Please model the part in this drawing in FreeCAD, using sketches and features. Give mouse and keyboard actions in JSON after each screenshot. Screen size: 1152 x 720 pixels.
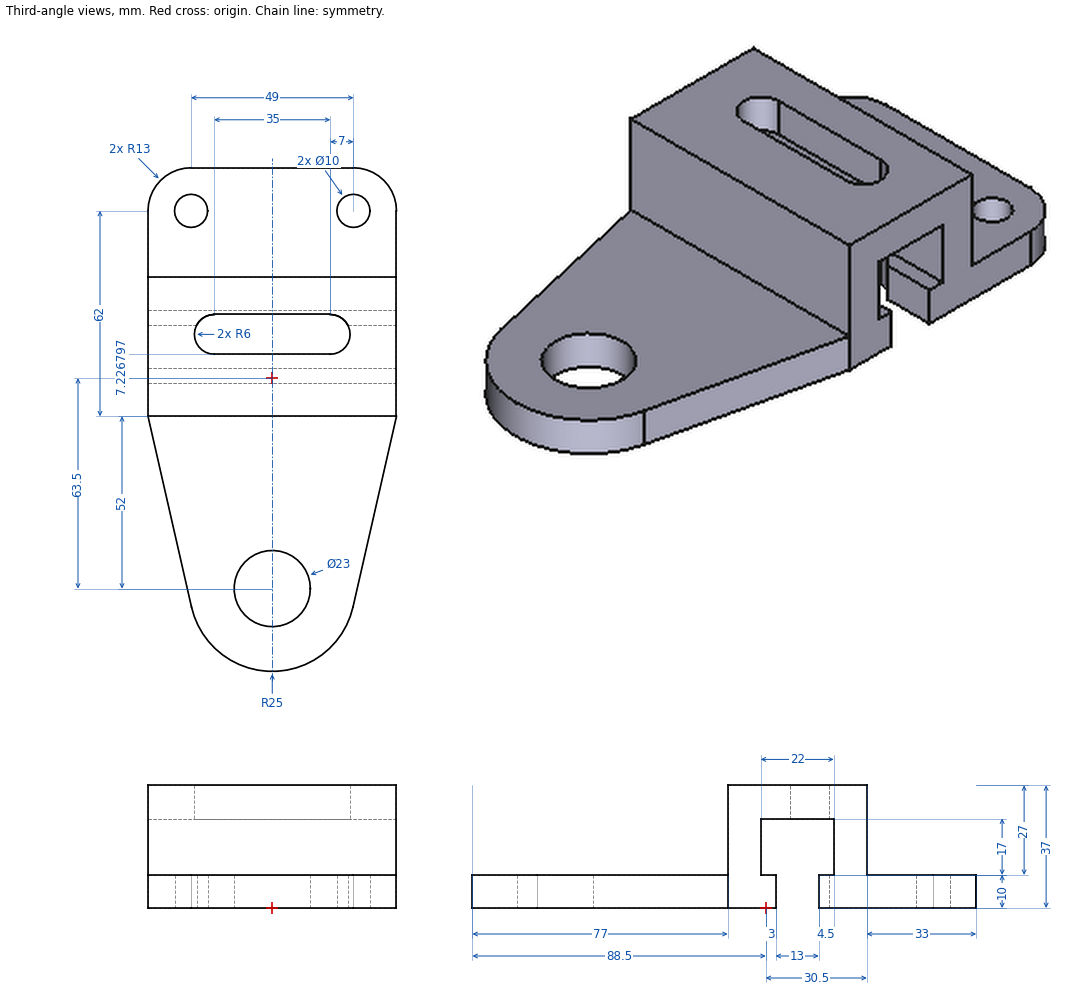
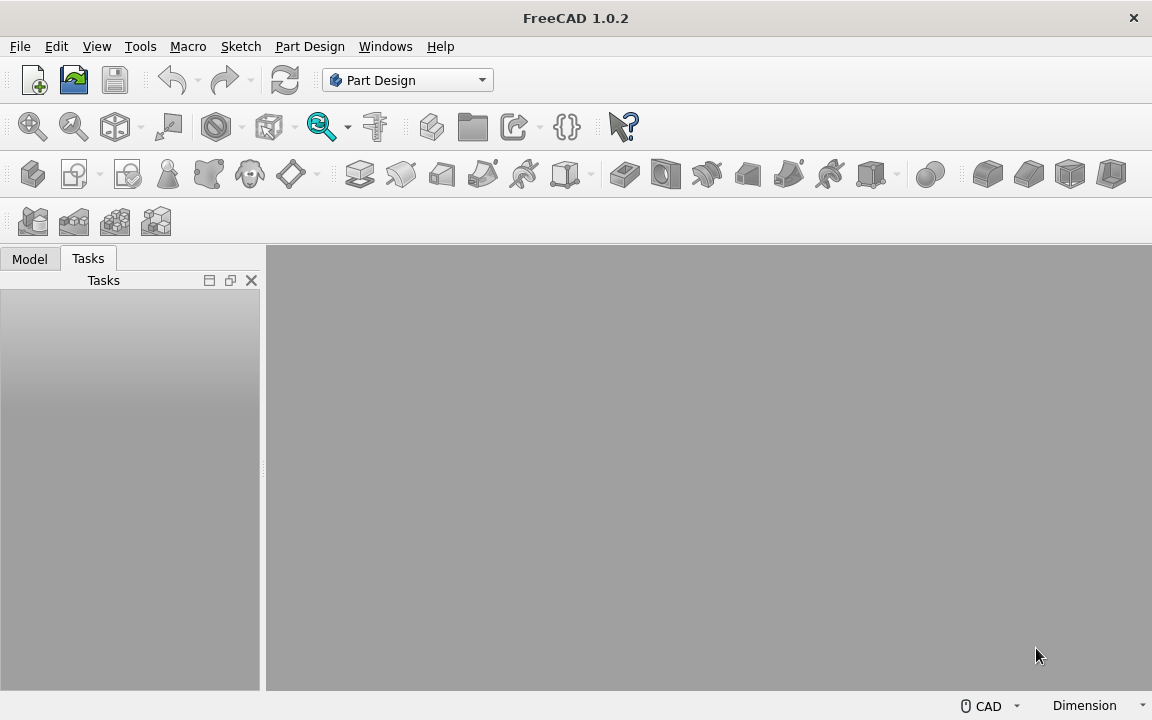
{"action": "left_click", "coordinate": [33, 80]}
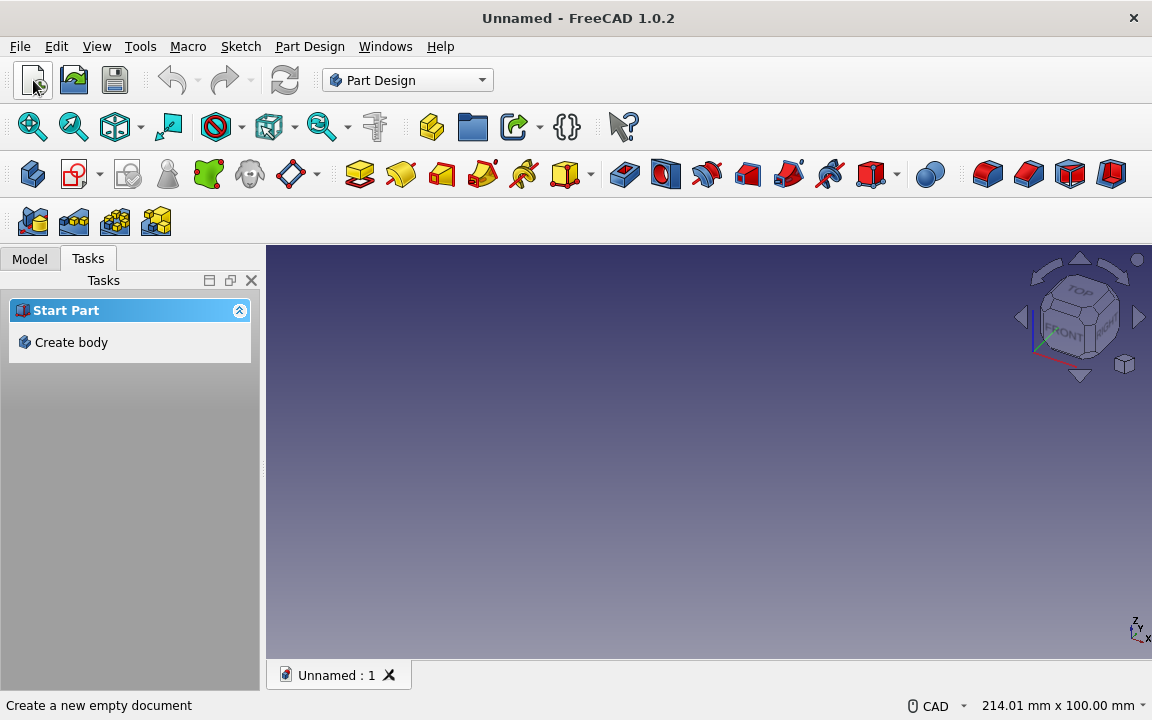
{"action": "left_click", "coordinate": [74, 174]}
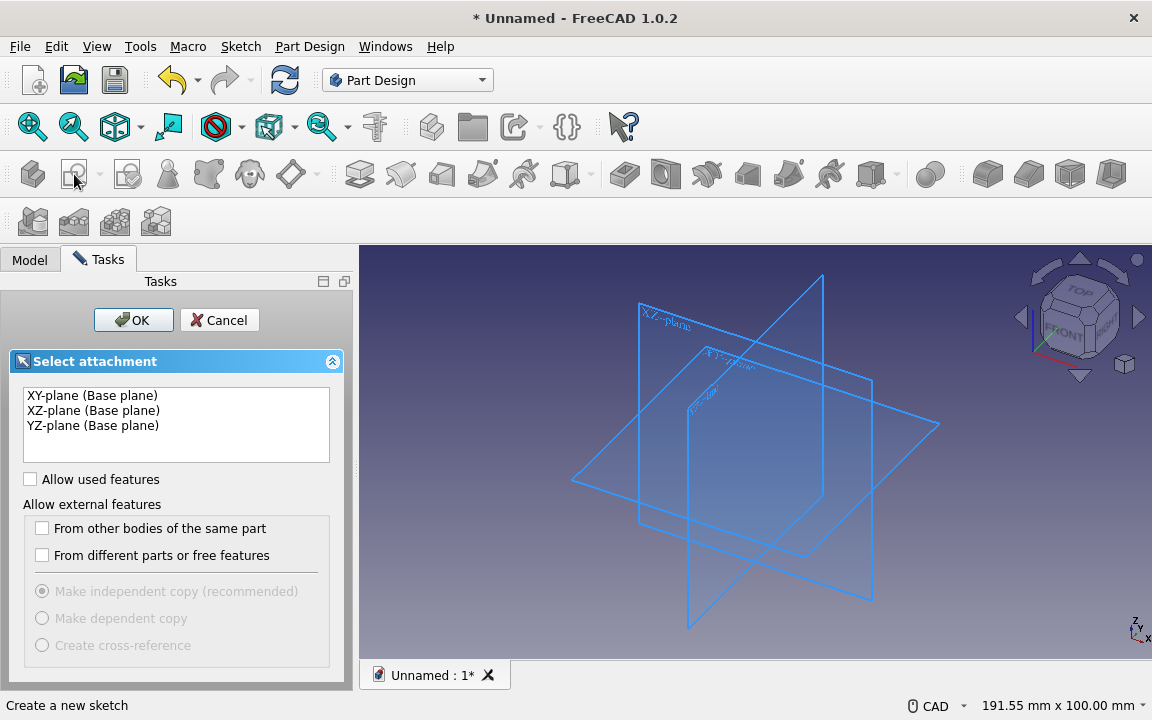
{"action": "left_click", "coordinate": [84, 396]}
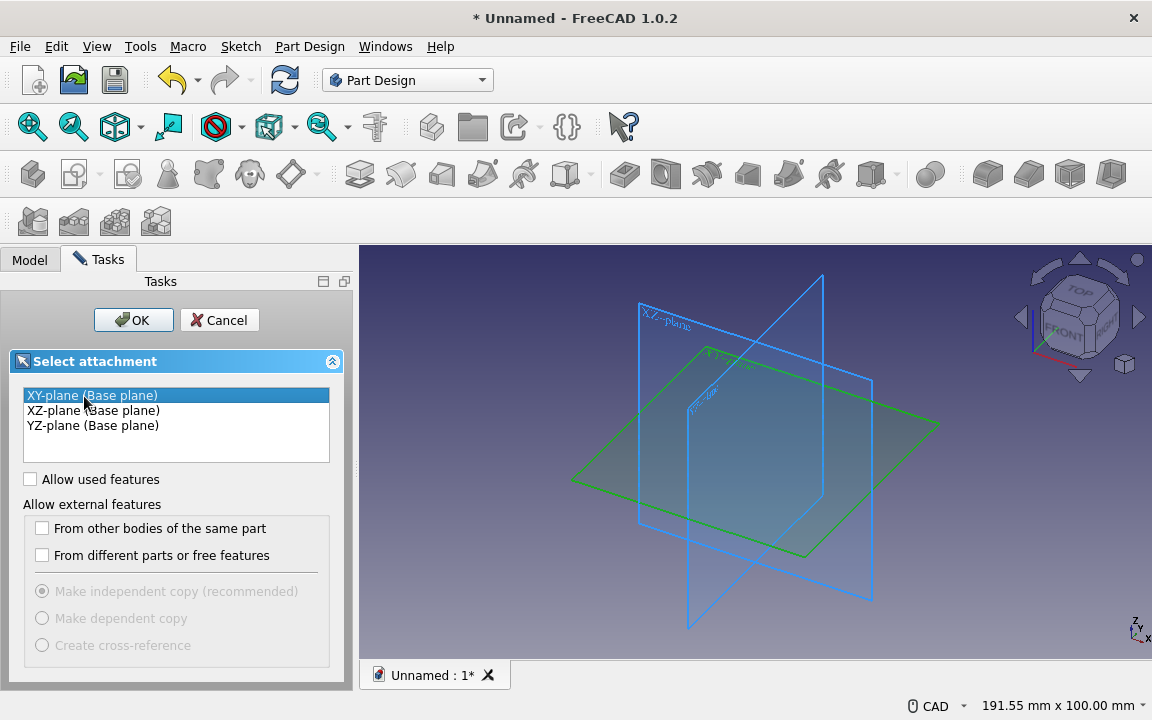
{"action": "left_click", "coordinate": [134, 320]}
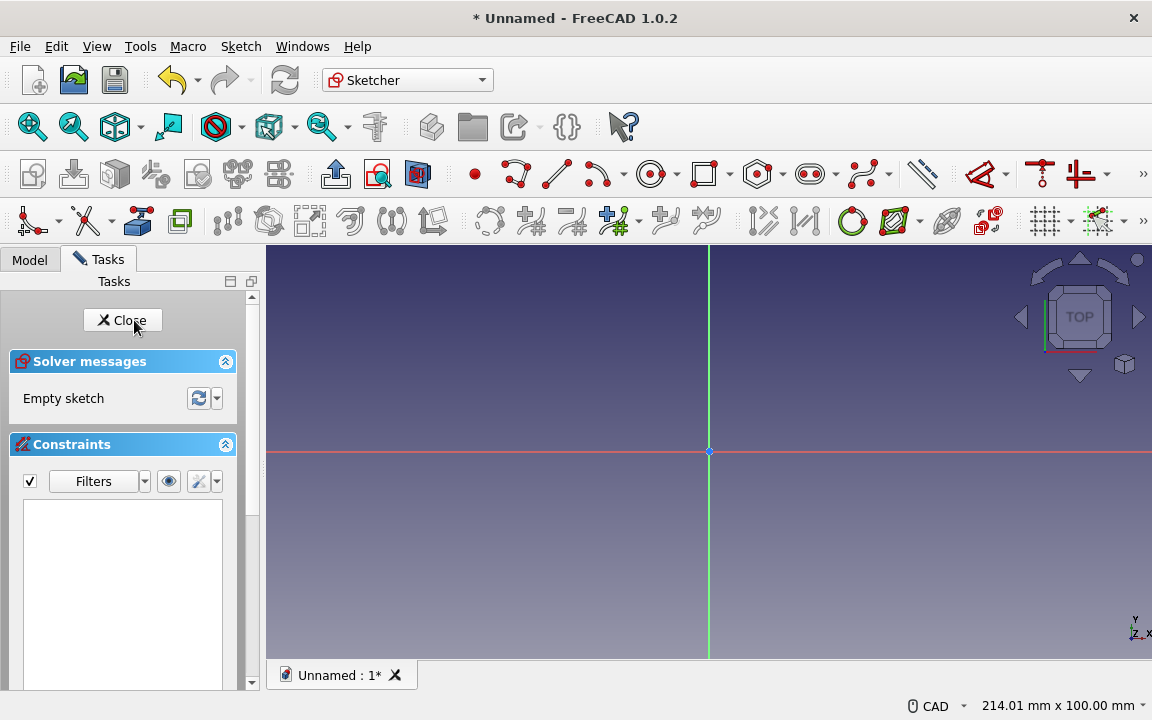
{"action": "scroll", "coordinate": [601, 422], "scroll_direction": "down", "scroll_amount": 5}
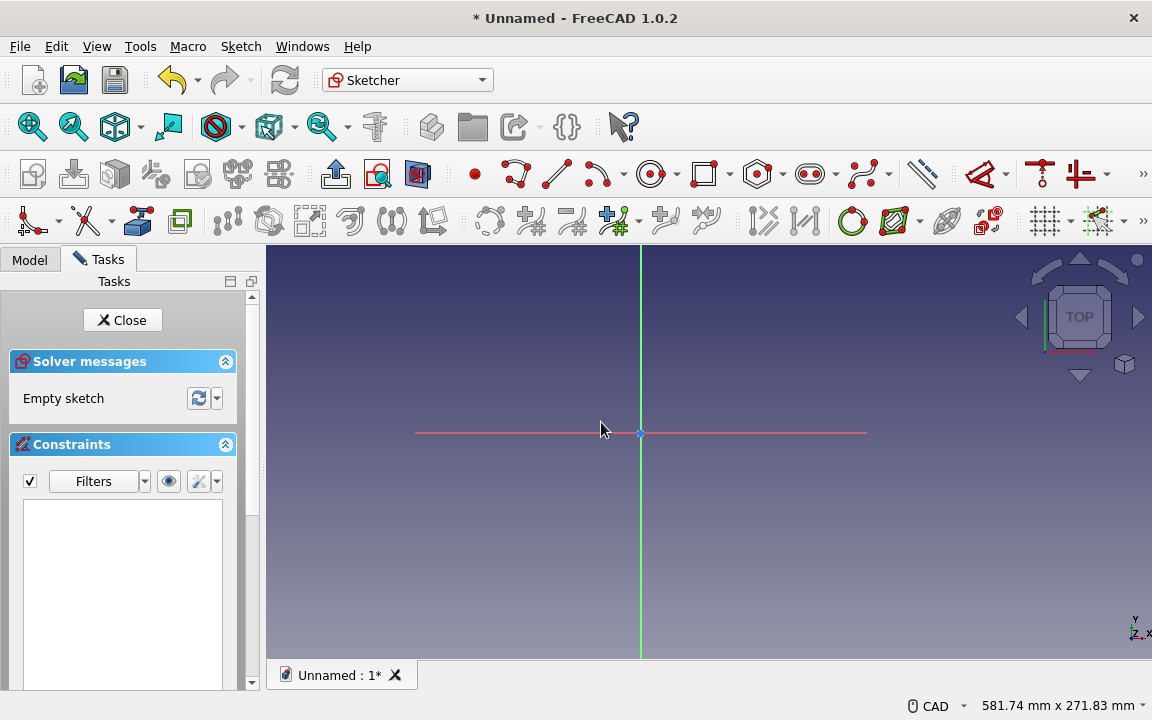
{"action": "left_click", "coordinate": [557, 174]}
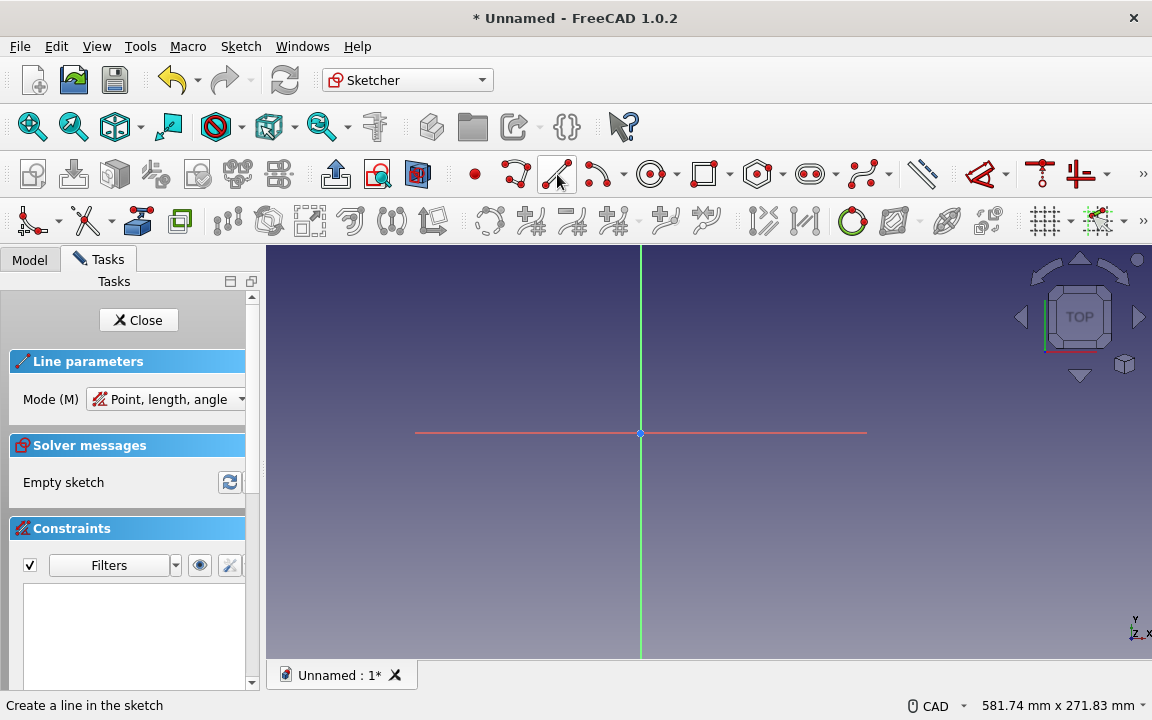
{"action": "left_click", "coordinate": [678, 337]}
{"action": "left_click", "coordinate": [604, 337]}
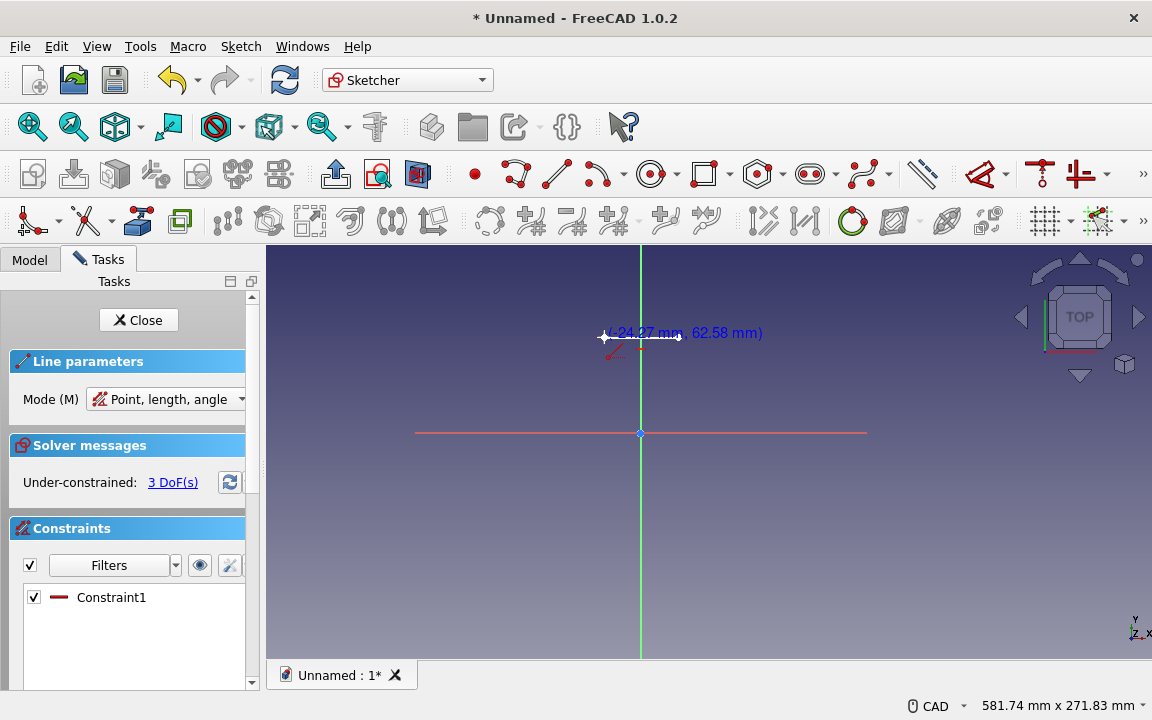
{"action": "left_click", "coordinate": [516, 174]}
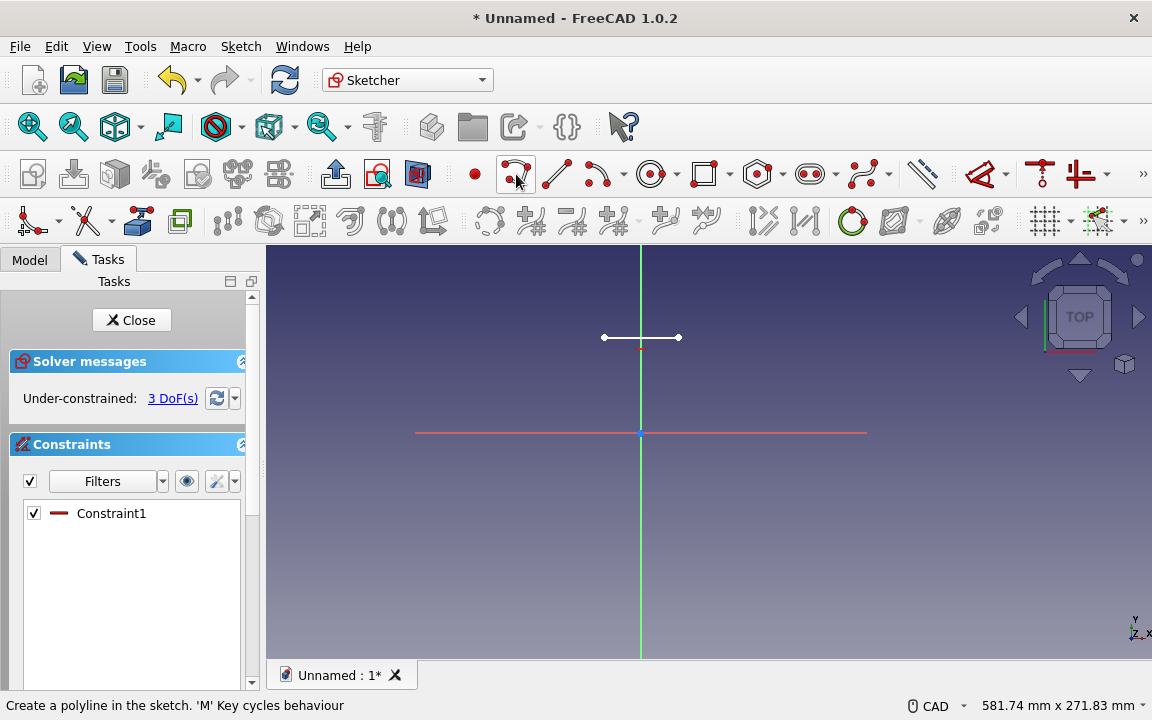
{"action": "left_click", "coordinate": [584, 356]}
{"action": "left_click", "coordinate": [584, 451]}
{"action": "left_click", "coordinate": [604, 538]}
{"action": "right_click", "coordinate": [604, 538]}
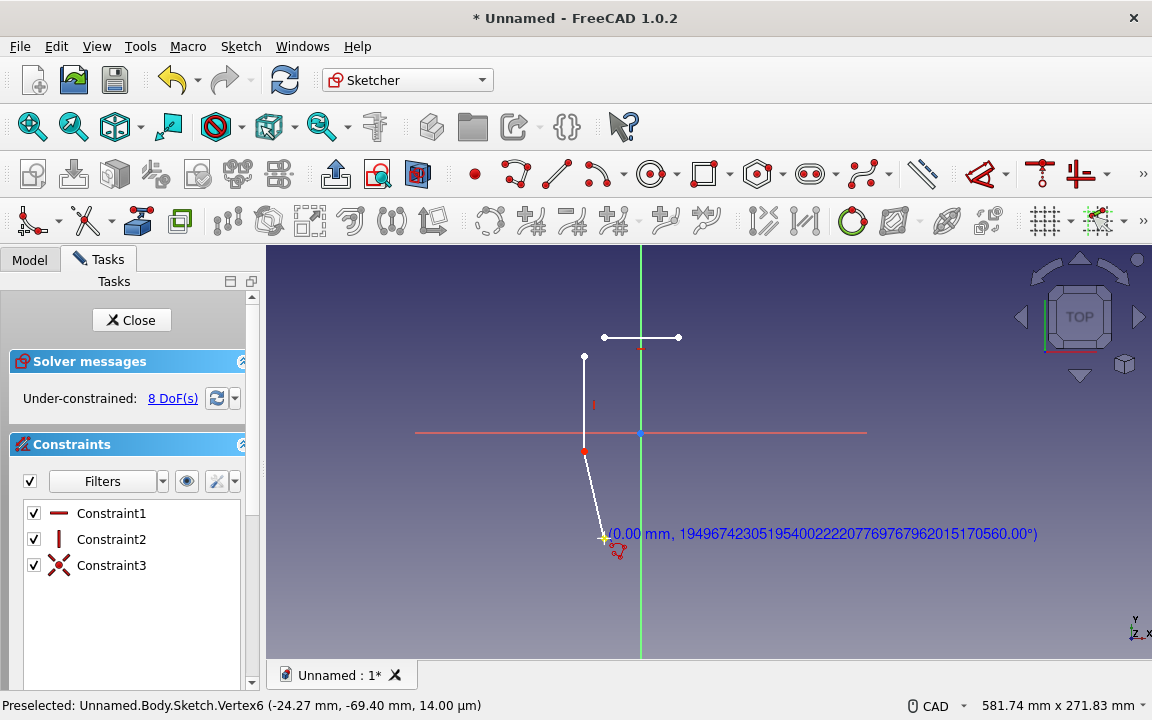
{"action": "left_click", "coordinate": [678, 538]}
{"action": "left_click", "coordinate": [698, 451]}
{"action": "left_click", "coordinate": [698, 356]}
{"action": "right_click", "coordinate": [698, 356]}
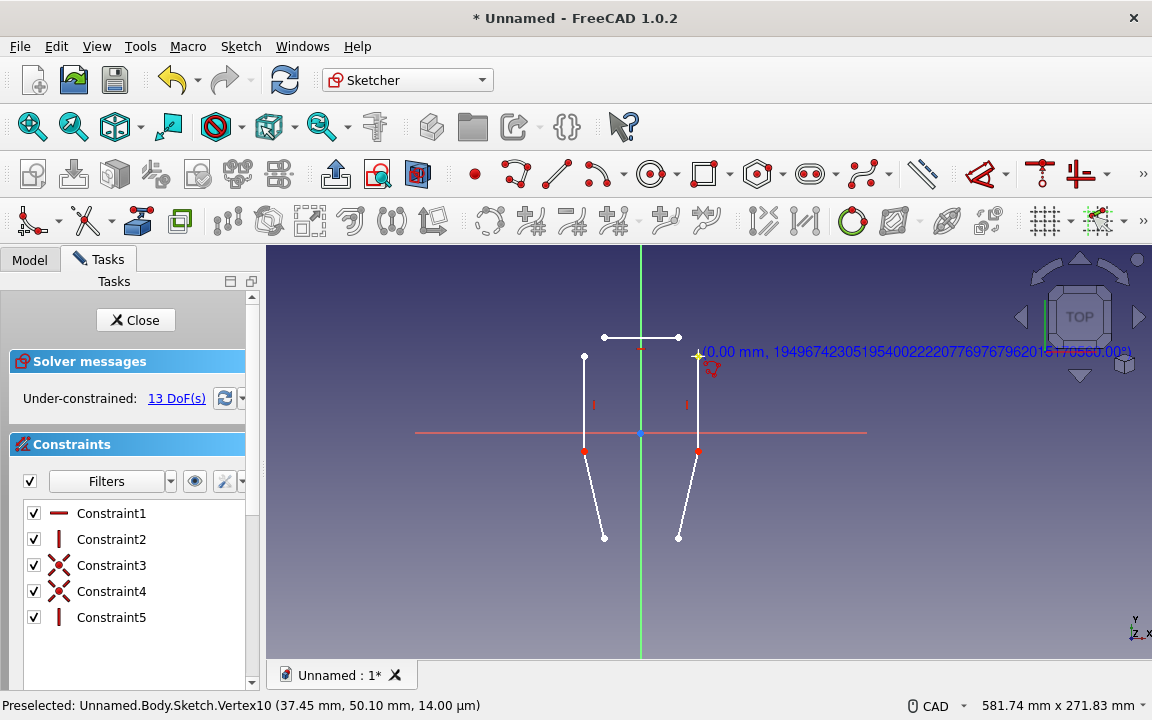
{"action": "left_click", "coordinate": [624, 174]}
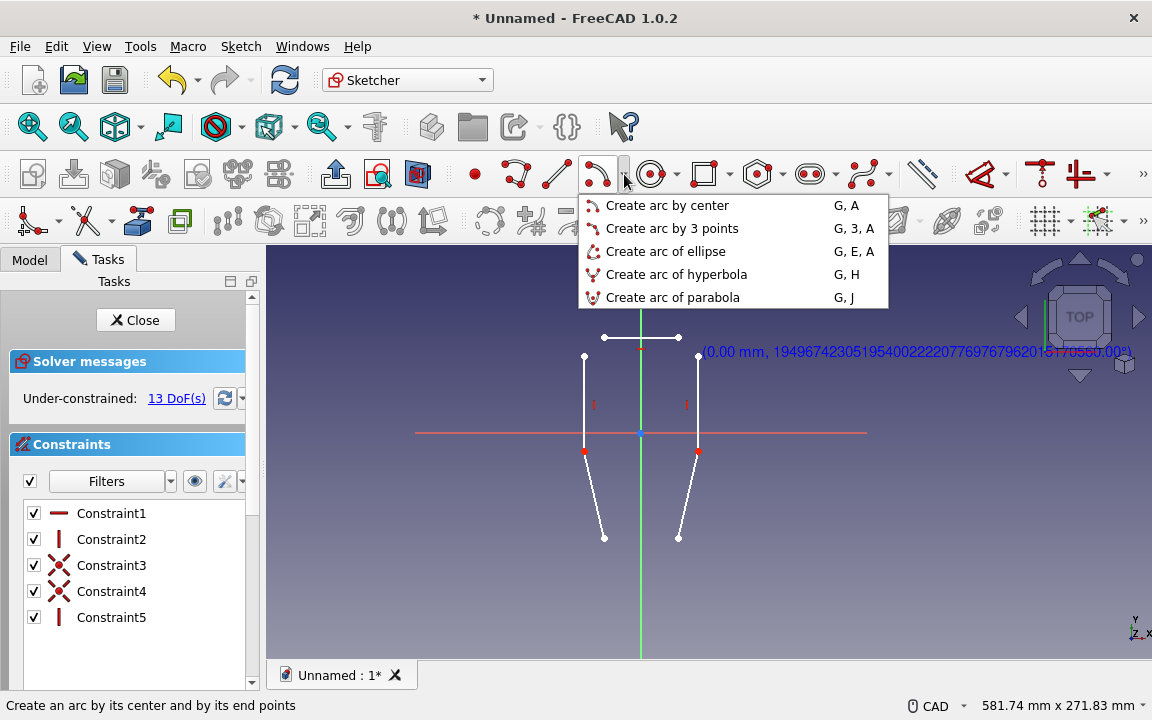
{"action": "left_click", "coordinate": [734, 228]}